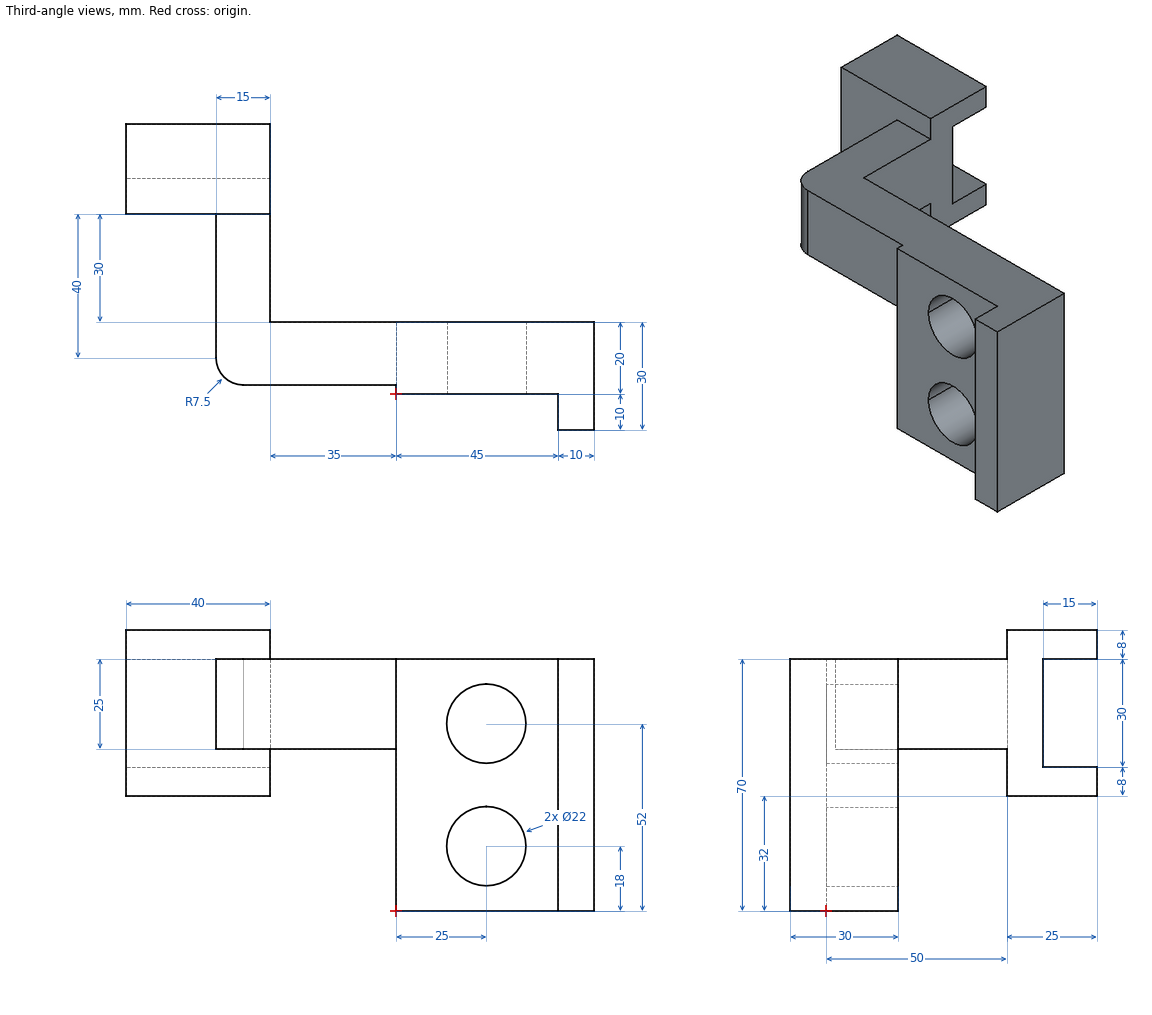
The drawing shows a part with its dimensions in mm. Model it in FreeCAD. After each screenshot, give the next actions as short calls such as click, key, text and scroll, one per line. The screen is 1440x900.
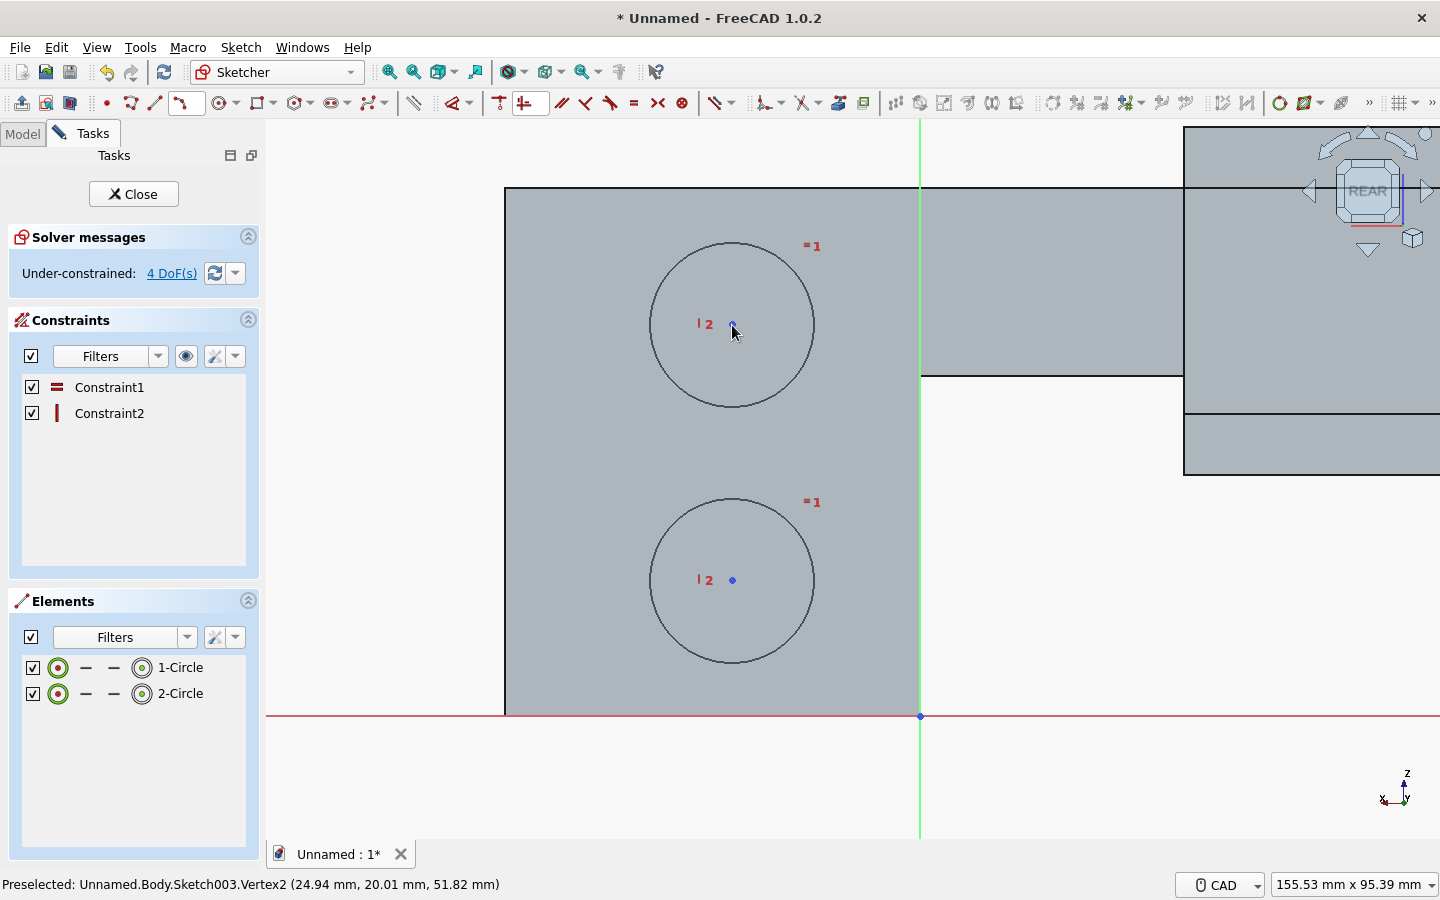
click(452, 104)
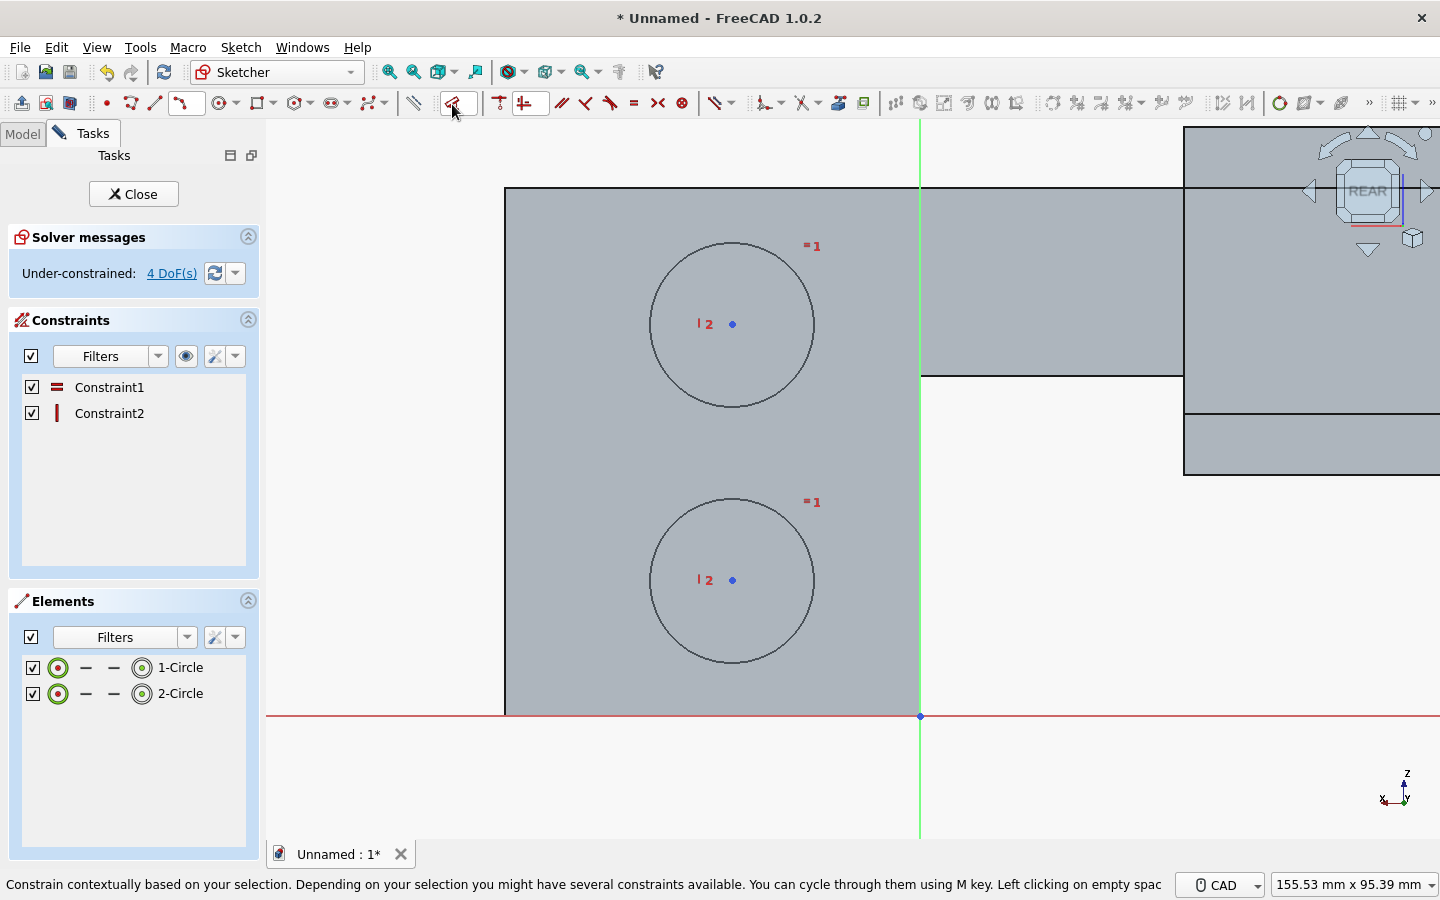
click(790, 523)
click(813, 500)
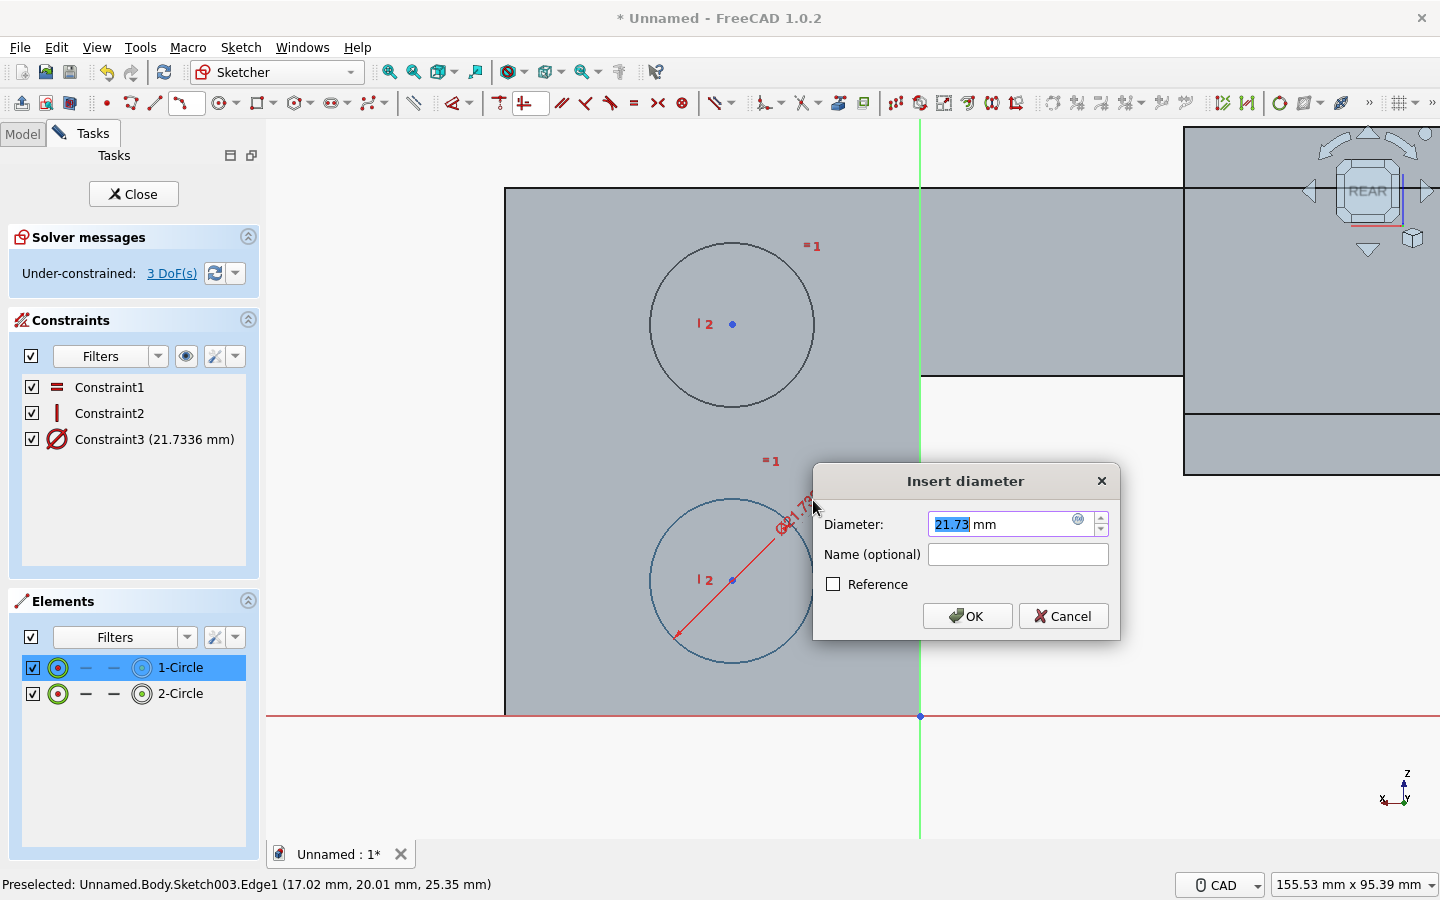
text(22)
key(Return)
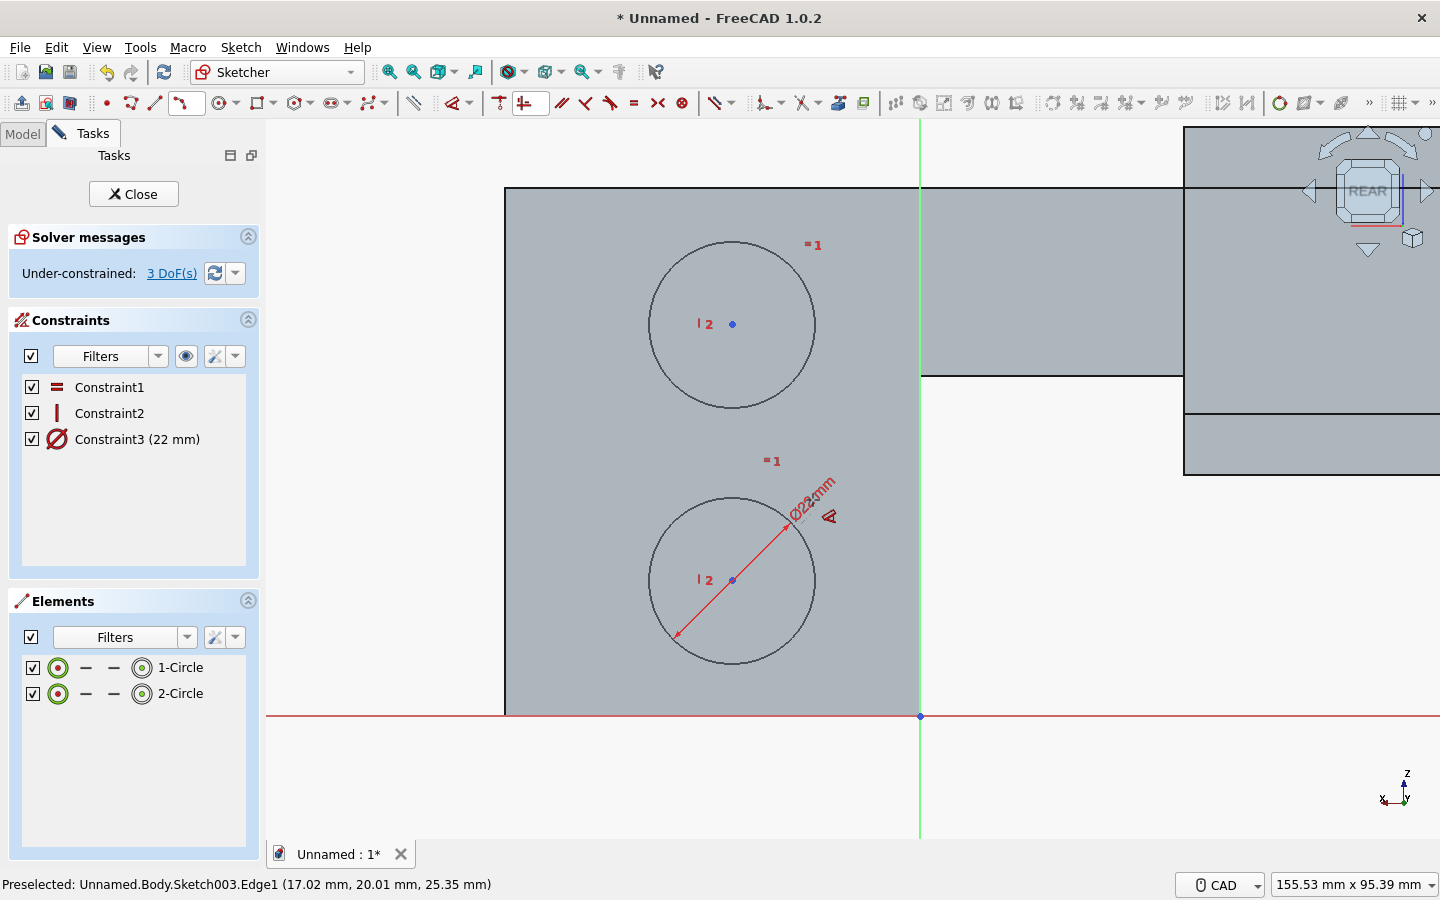
click(732, 581)
click(826, 750)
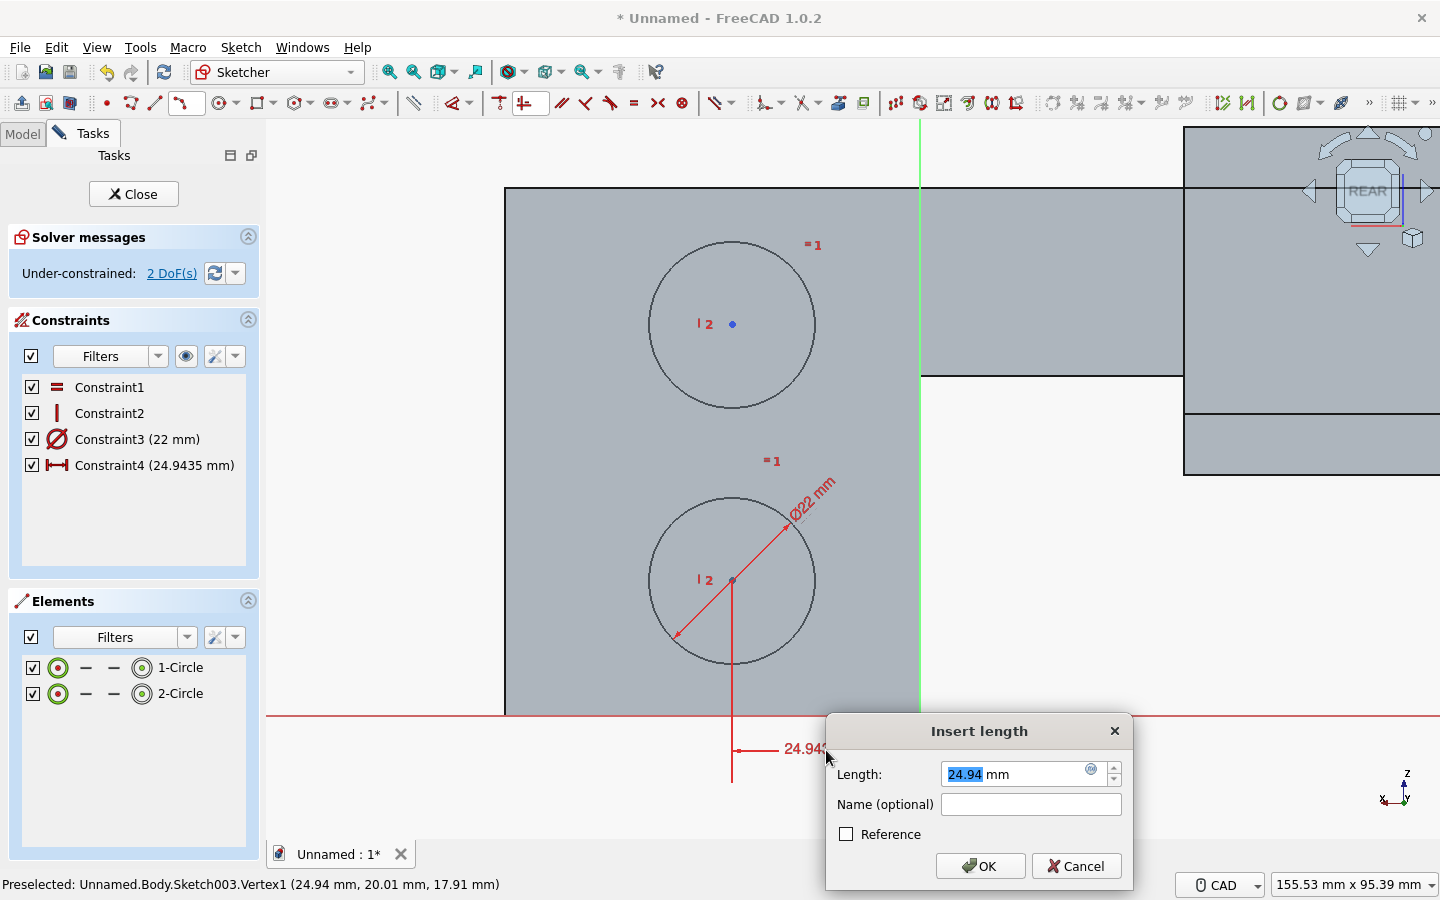
text(25)
key(Return)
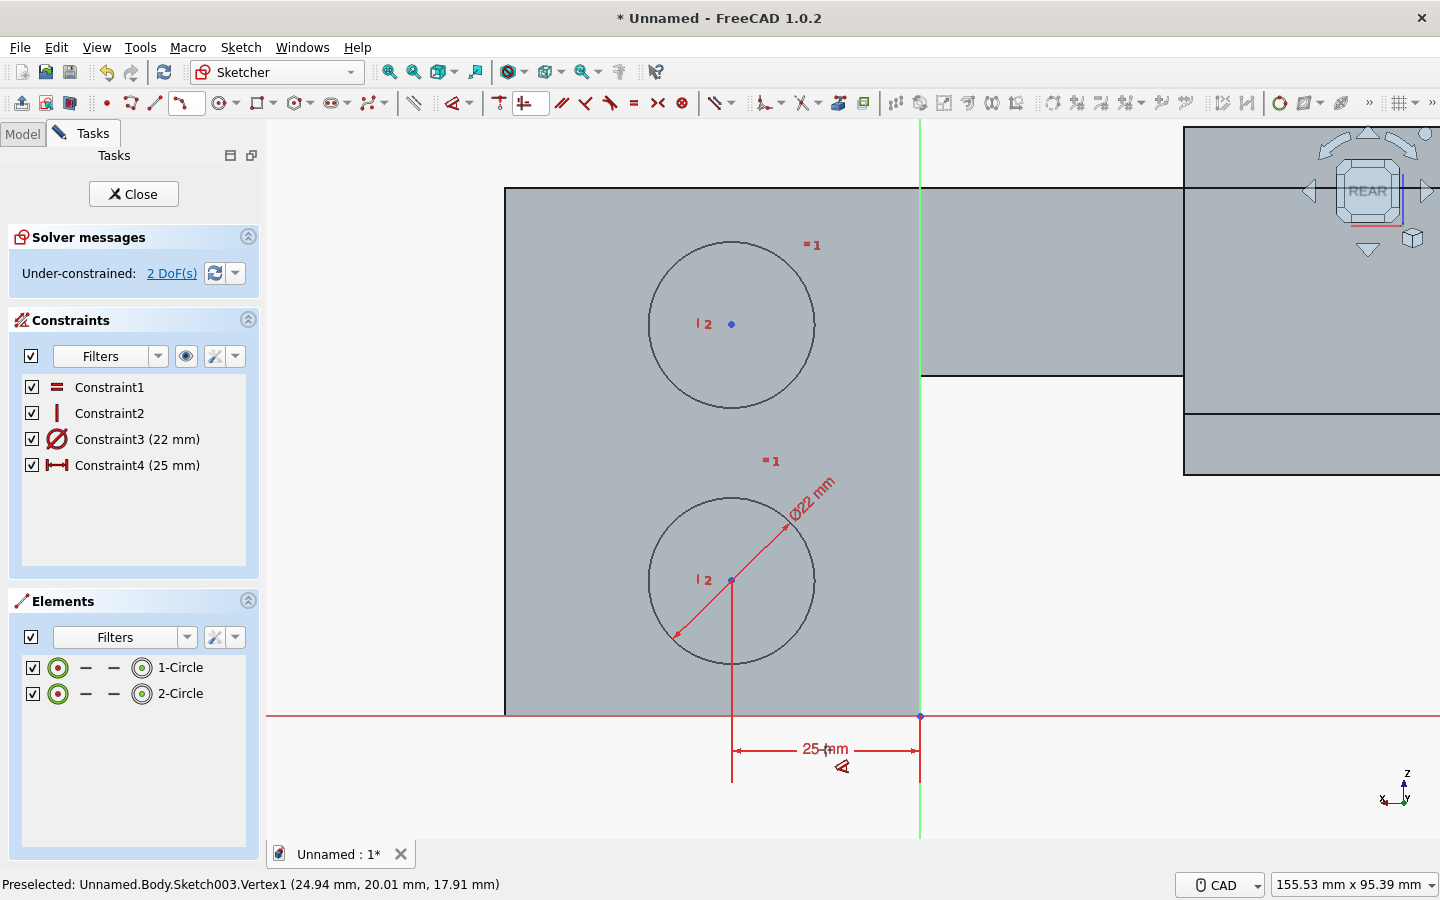
click(732, 581)
click(954, 649)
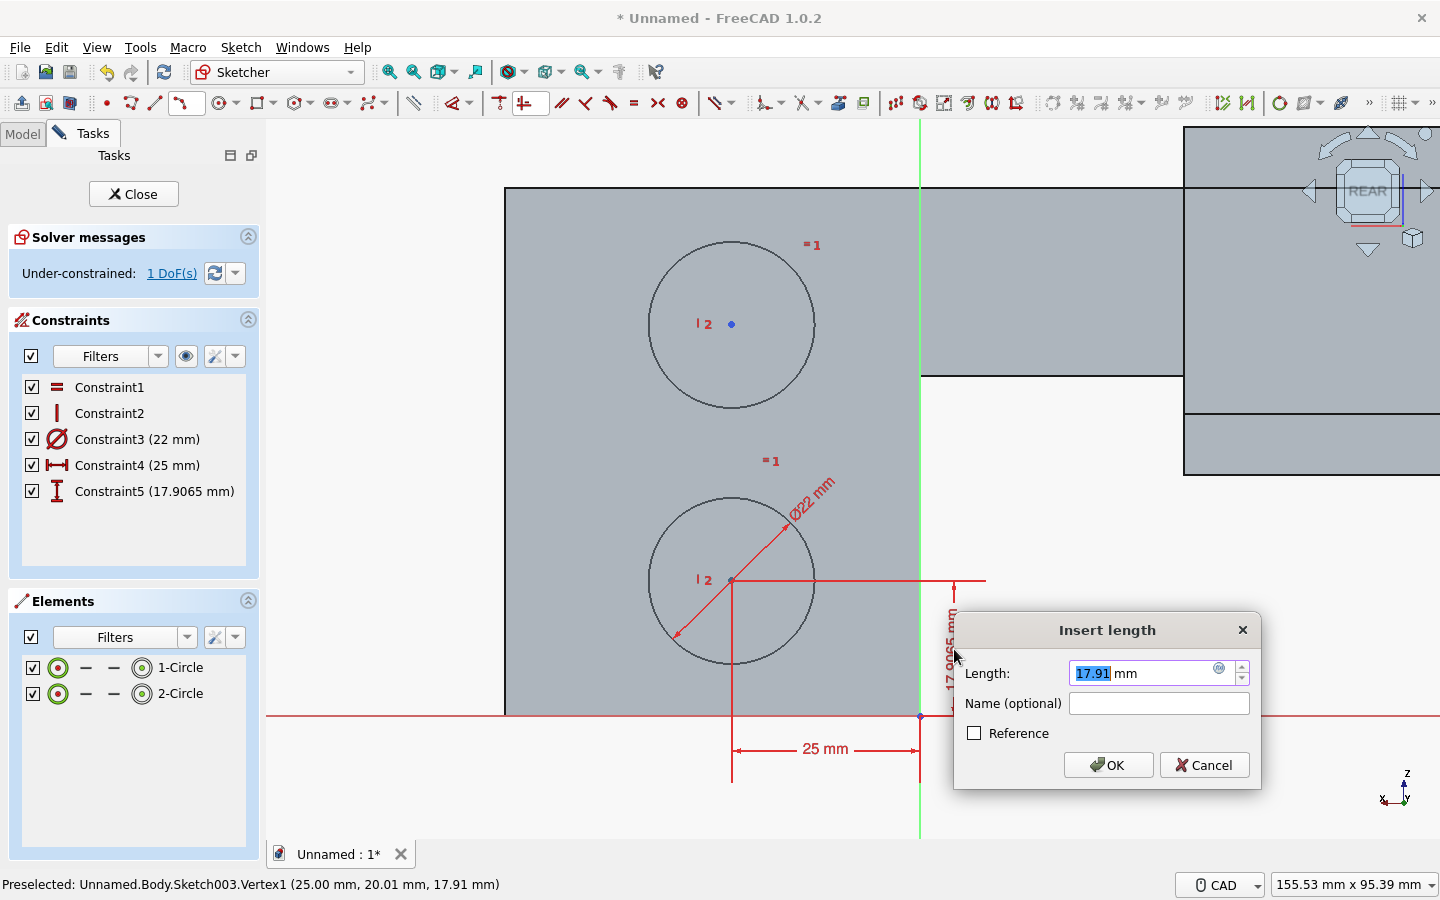
text(18)
key(Return)